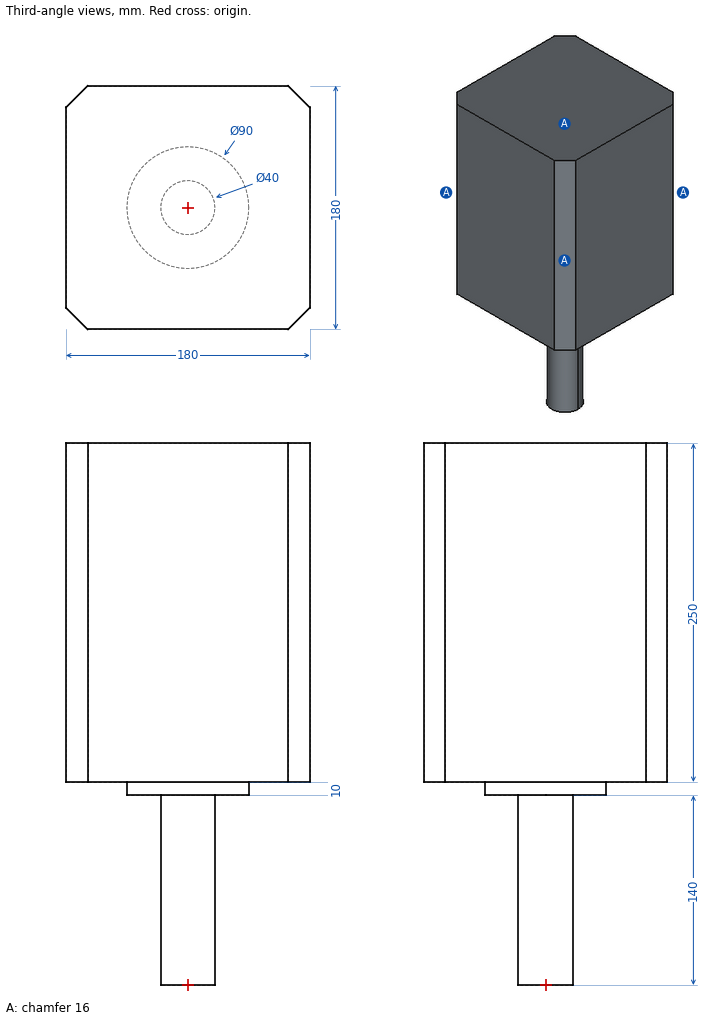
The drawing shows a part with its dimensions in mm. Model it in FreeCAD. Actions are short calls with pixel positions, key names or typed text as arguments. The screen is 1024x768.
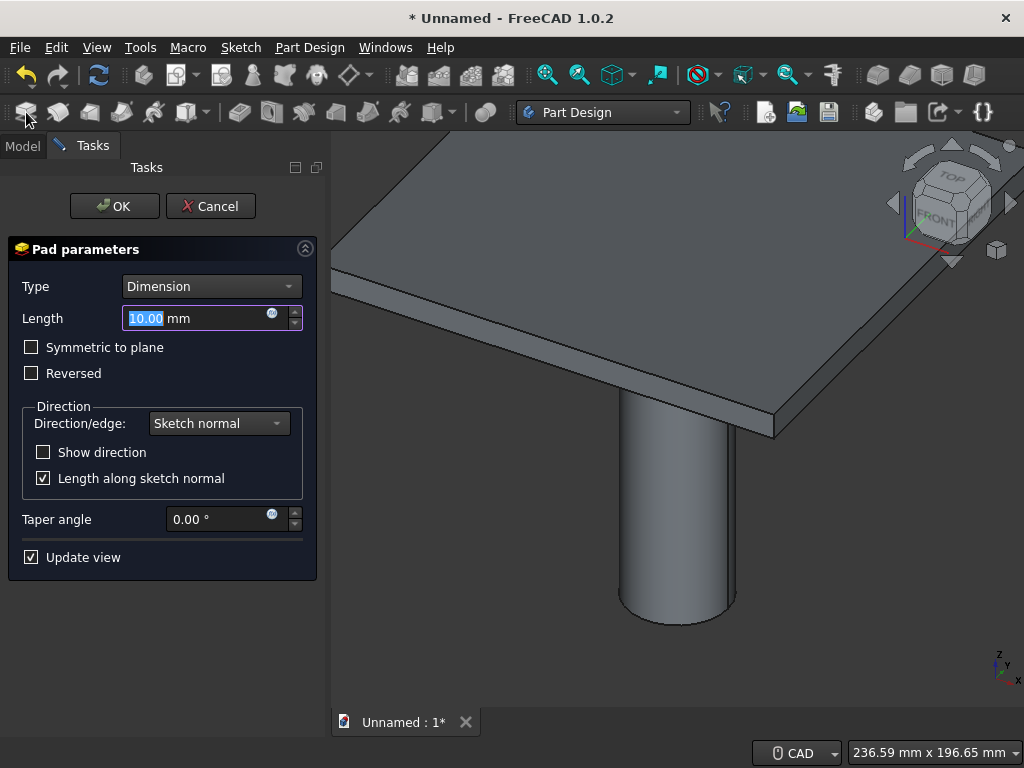
text(250)
key(Tab)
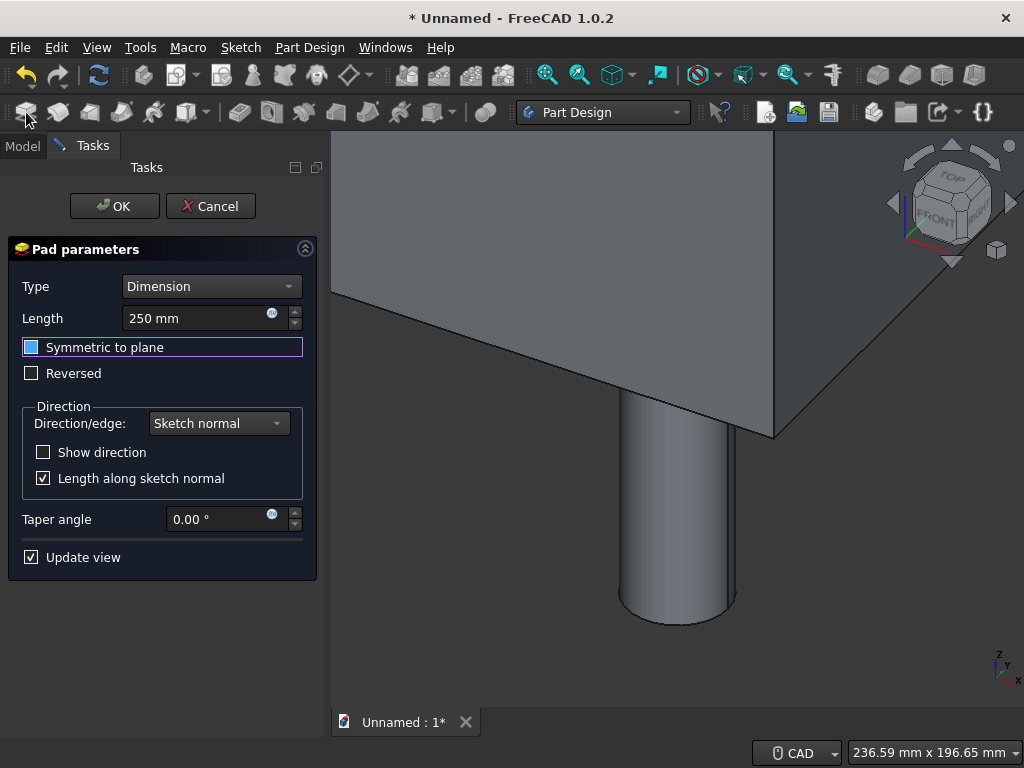
click(115, 206)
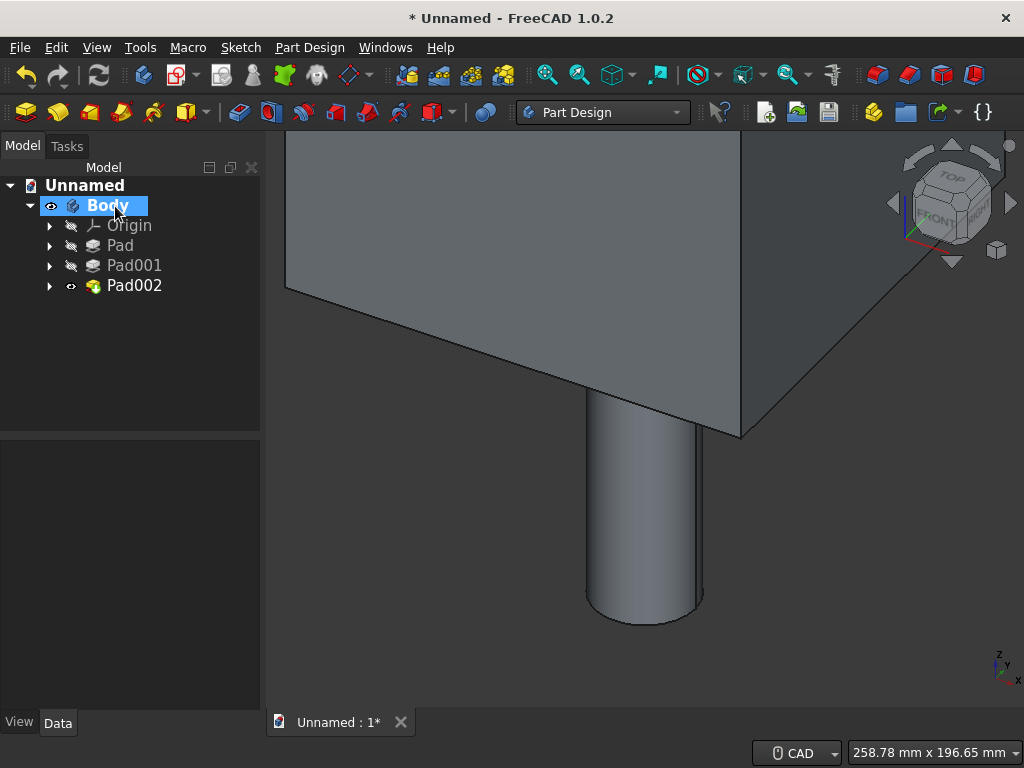
click(548, 76)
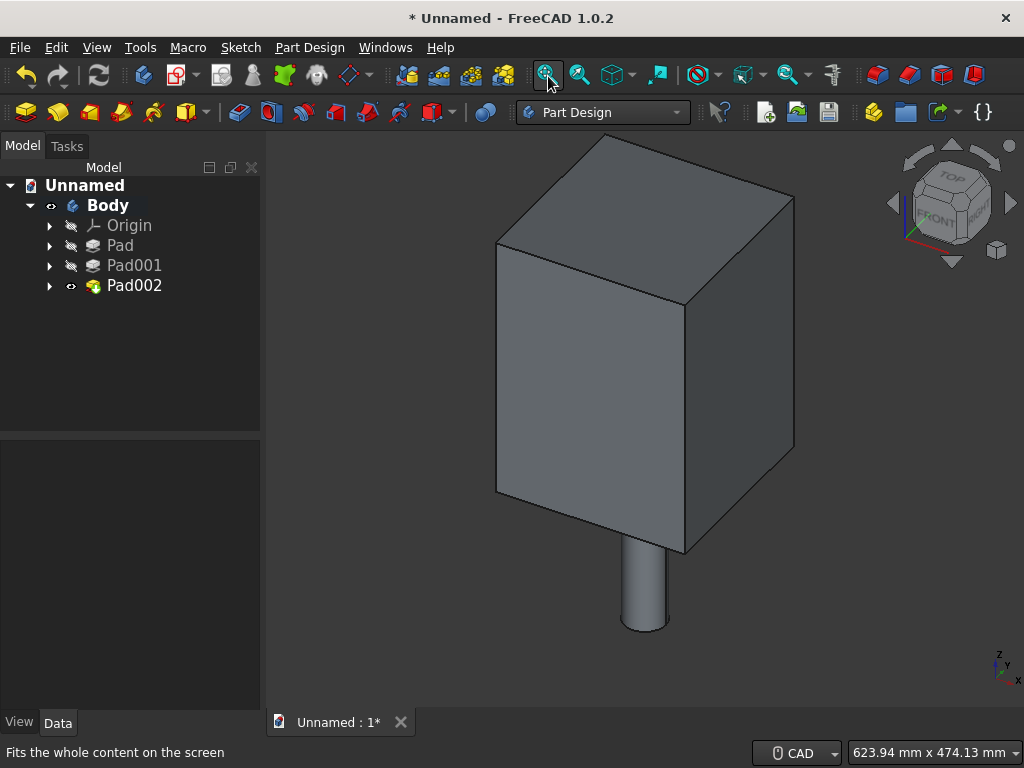
click(685, 429)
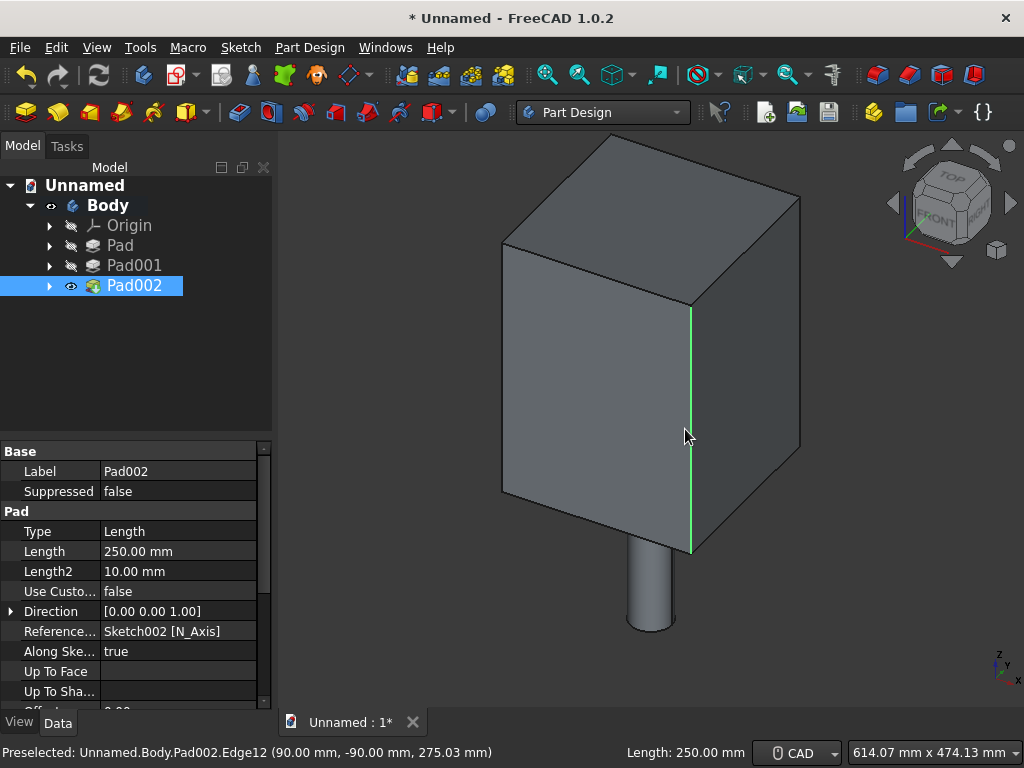
key(0)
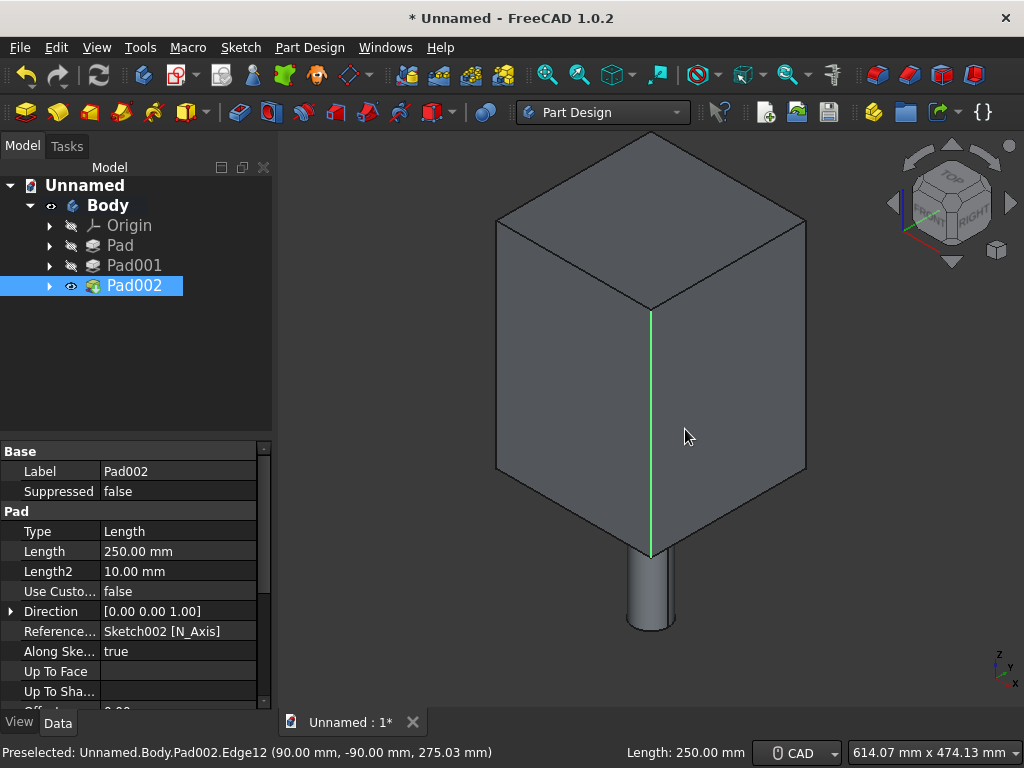
key(v)
key(f)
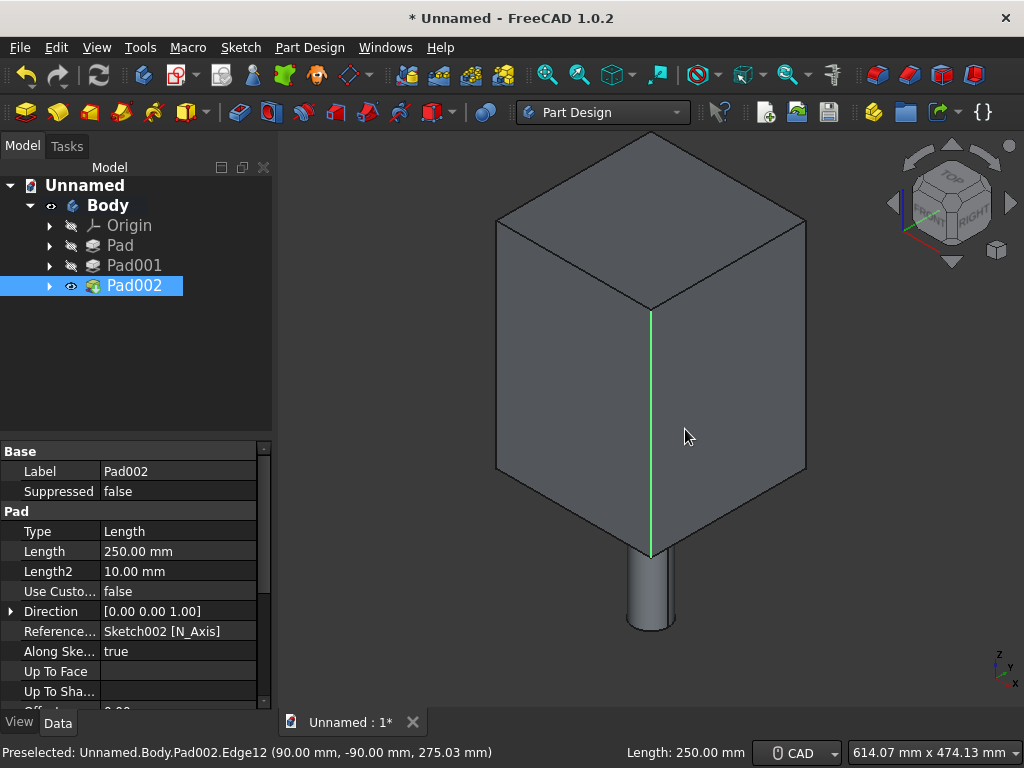
key(2)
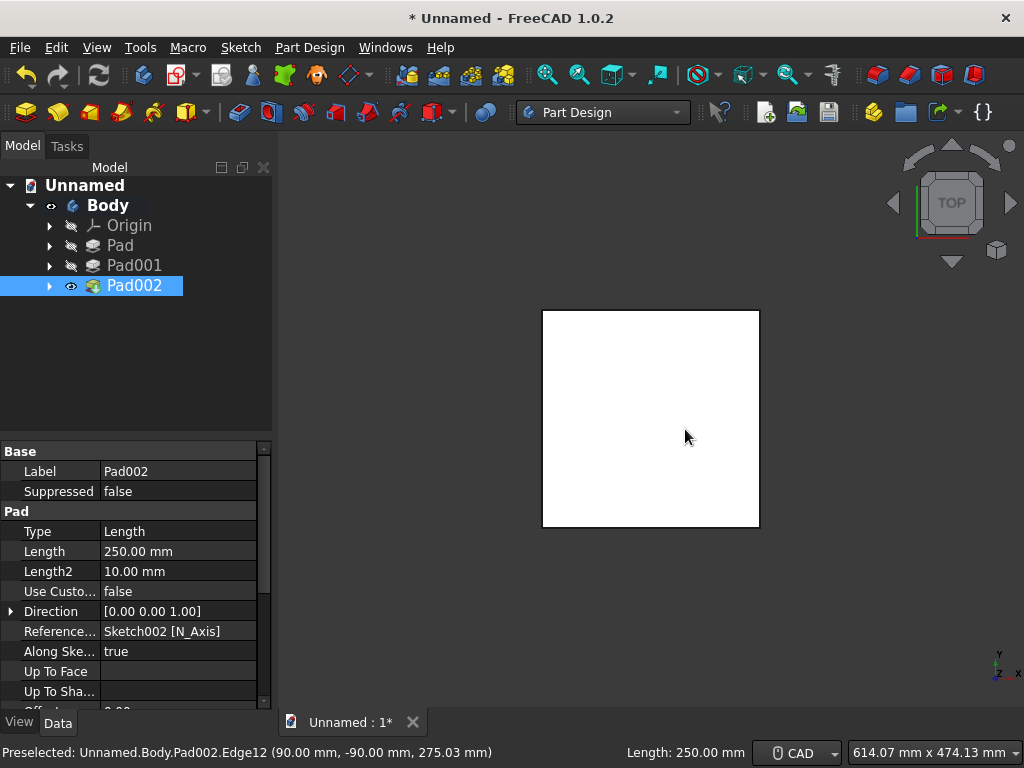
key(v)
key(f)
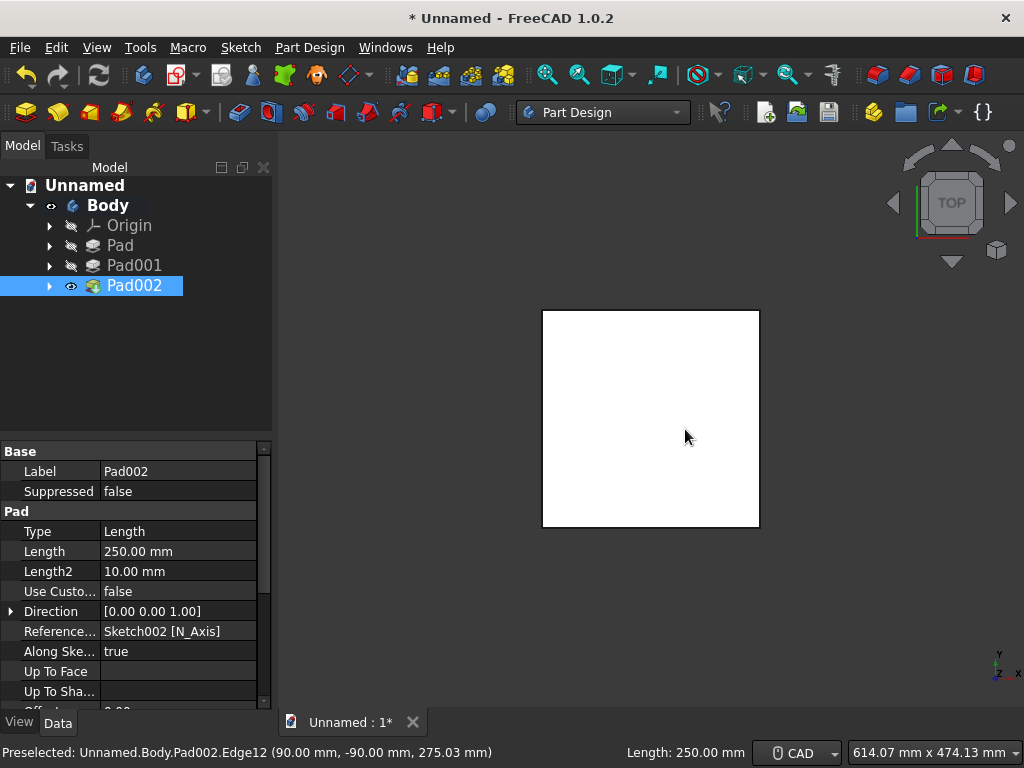
key(1)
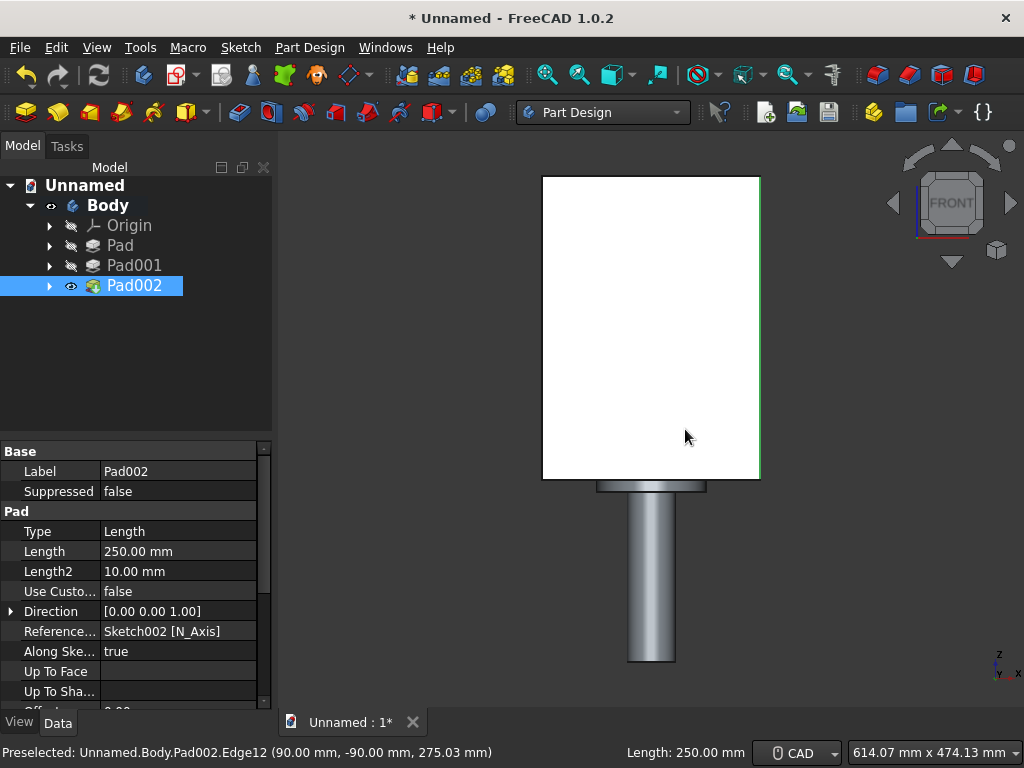
click(542, 327, ctrl)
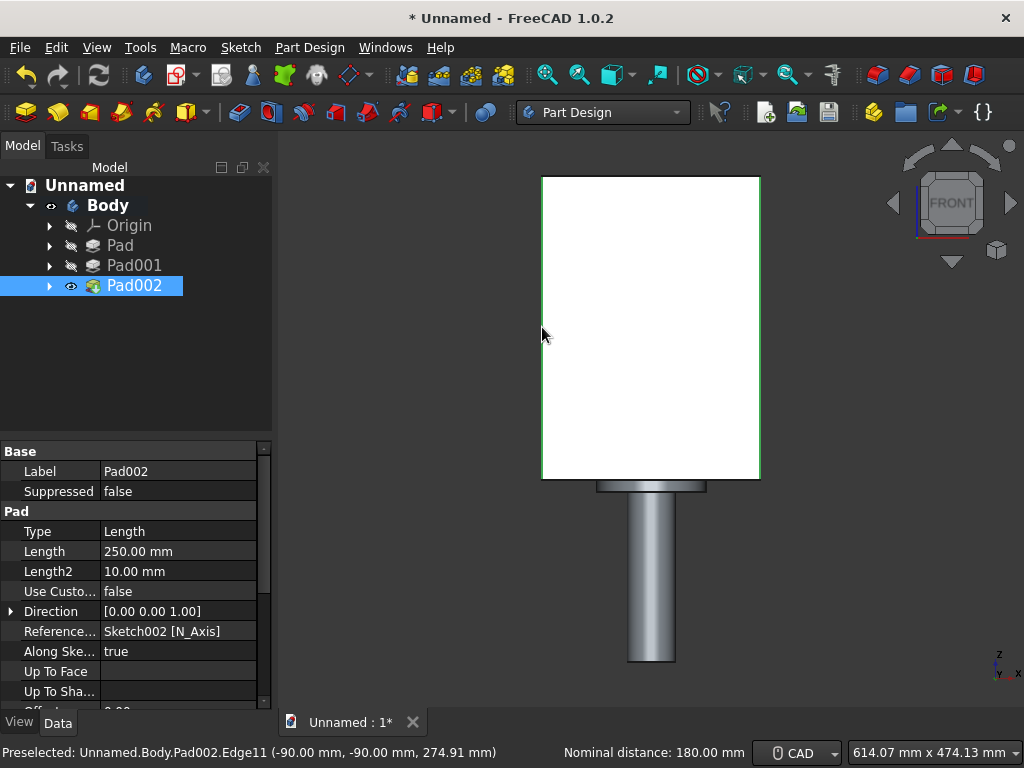
key(3)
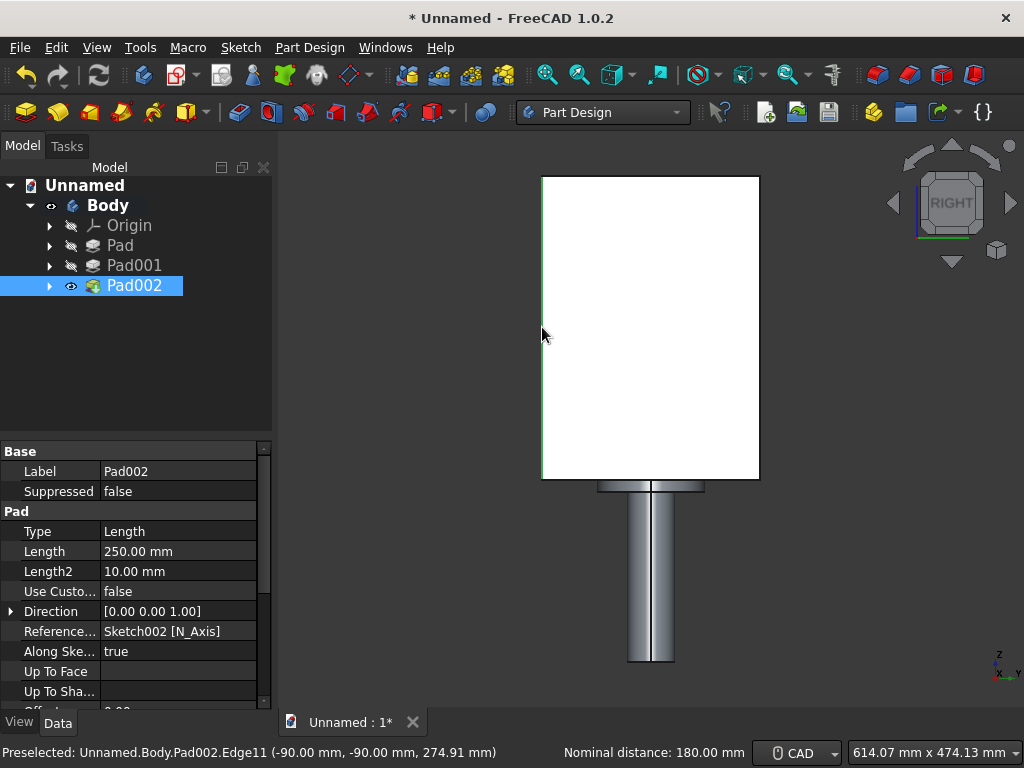
click(760, 327, ctrl)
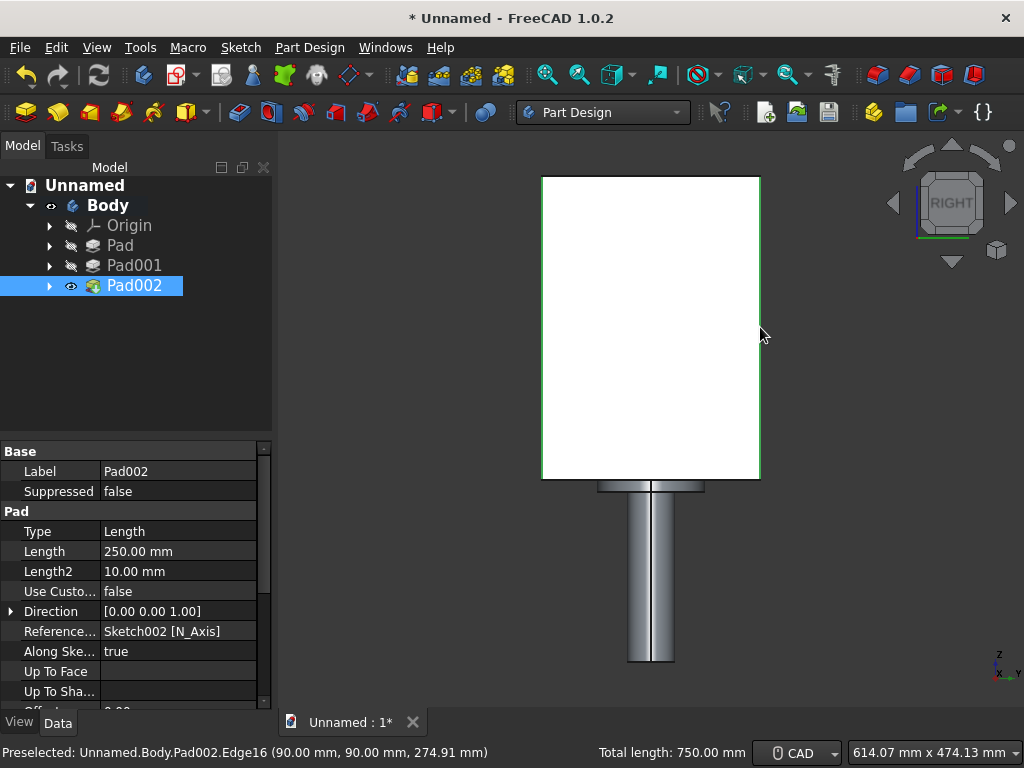
key(5)